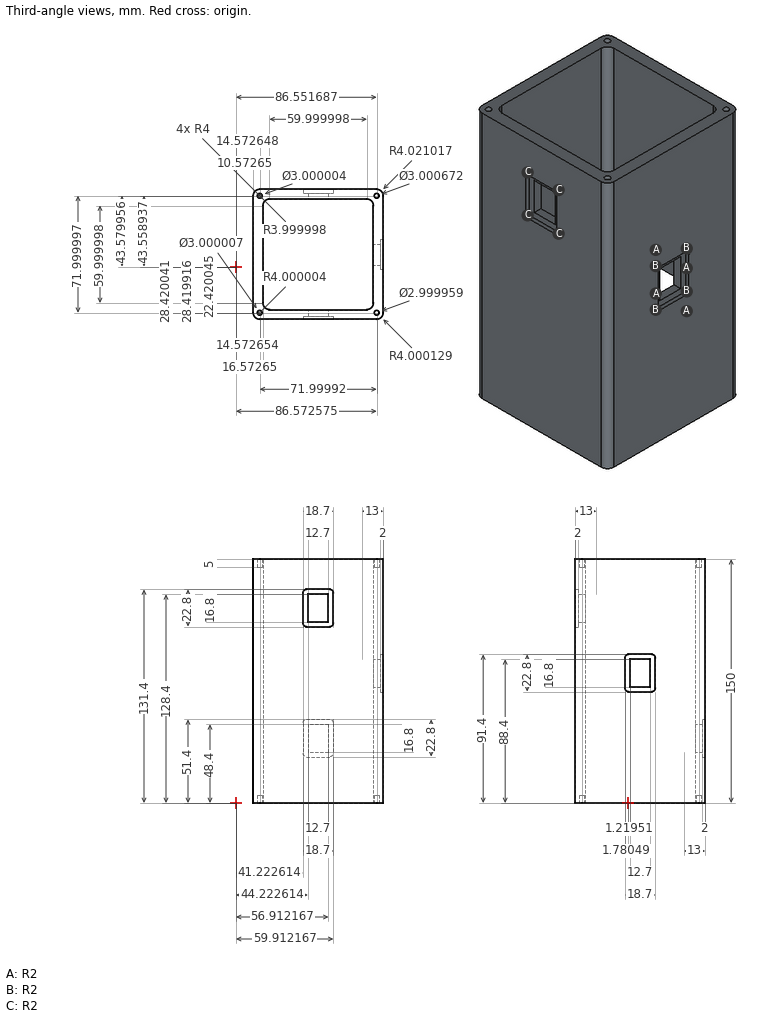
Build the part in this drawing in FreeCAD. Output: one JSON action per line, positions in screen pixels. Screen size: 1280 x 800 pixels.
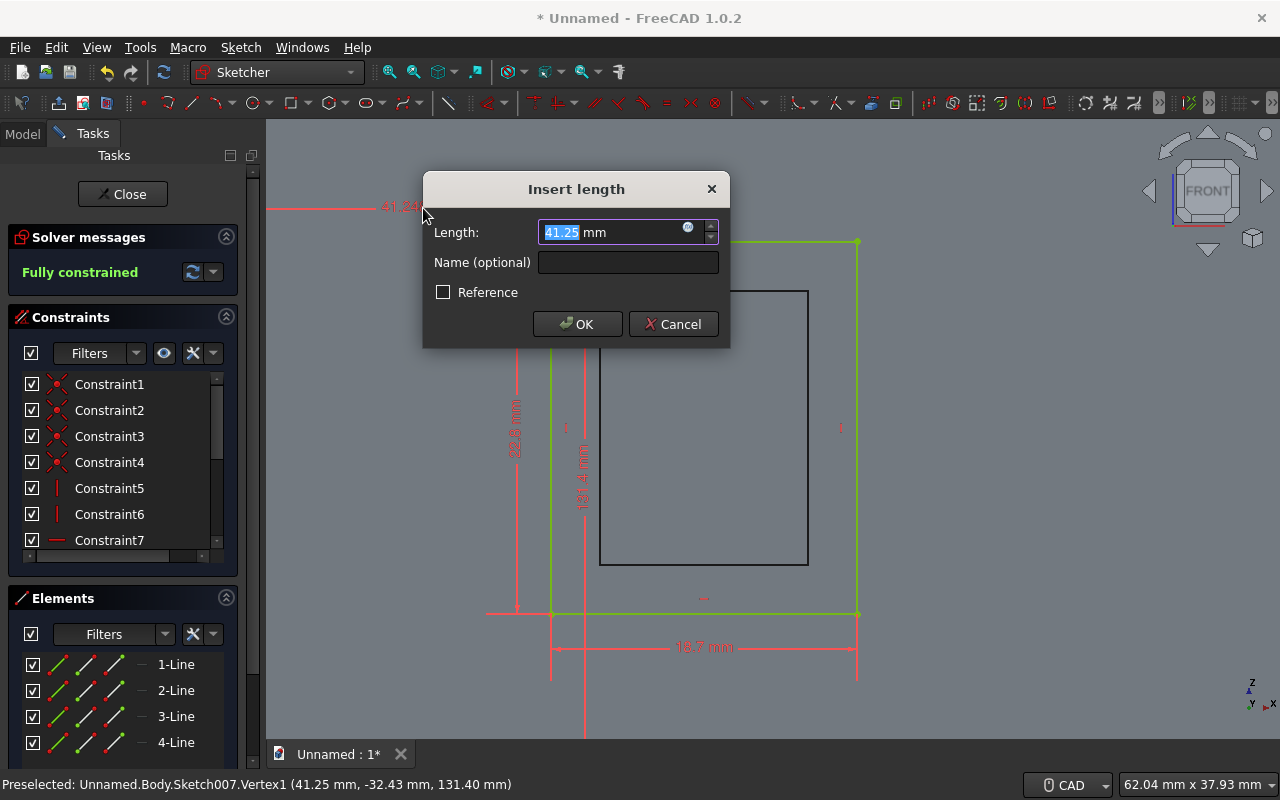
{"action": "type", "text": "41.222614"}
{"action": "key", "text": "Return"}
{"action": "key", "text": "Escape"}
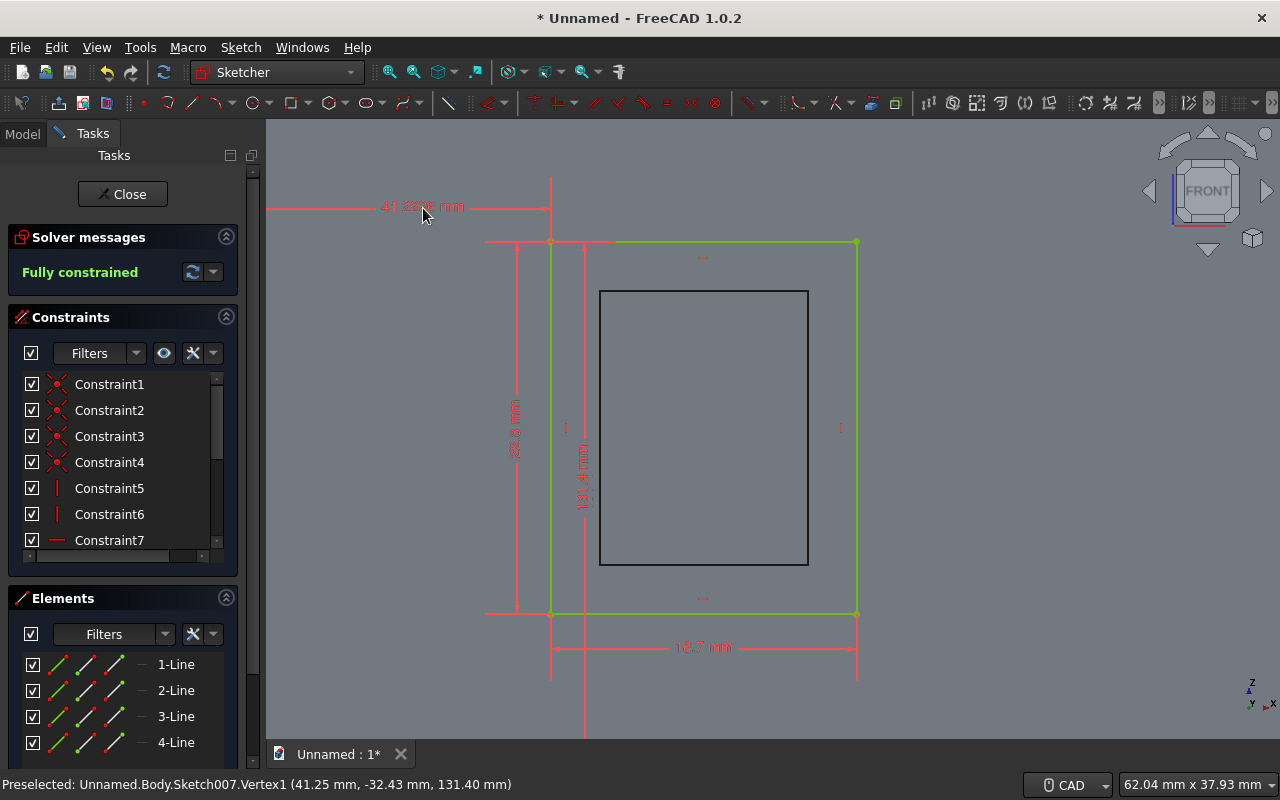
{"action": "left_click", "coordinate": [123, 194]}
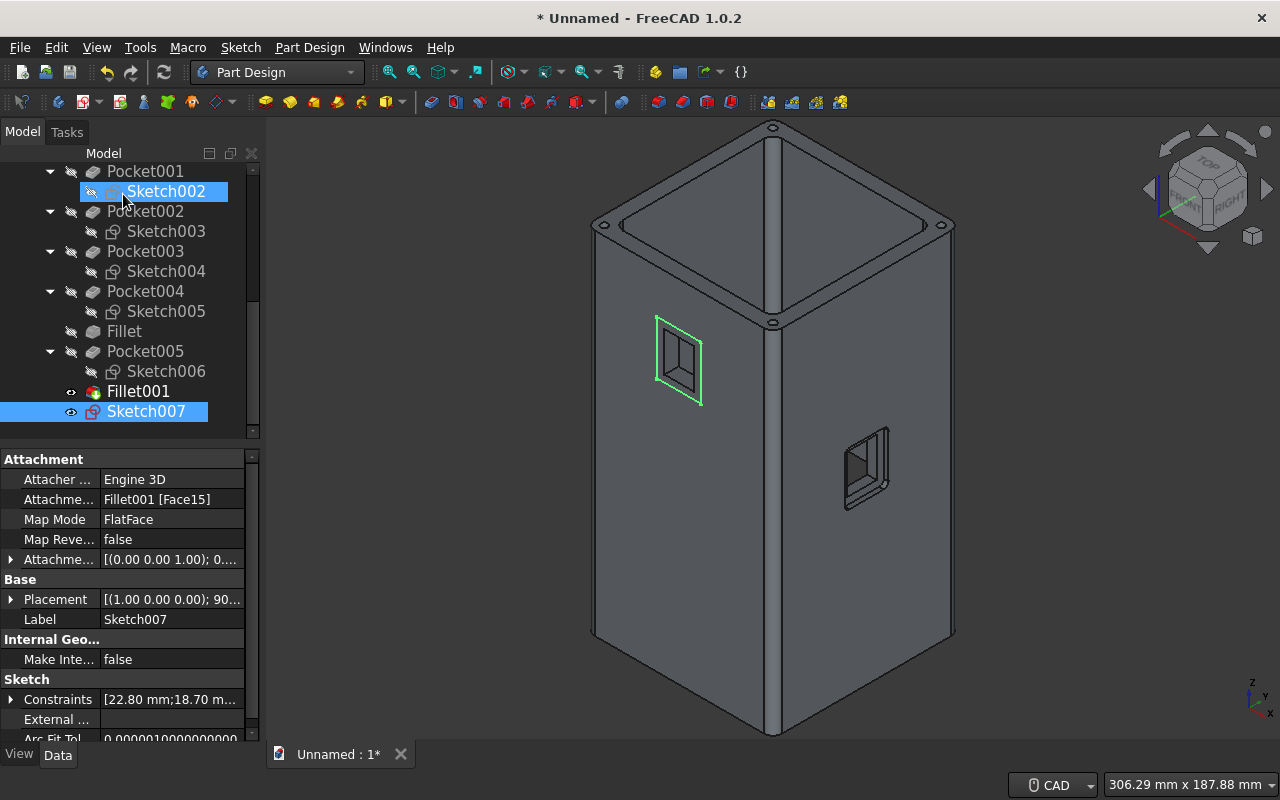
{"action": "left_click", "coordinate": [432, 102]}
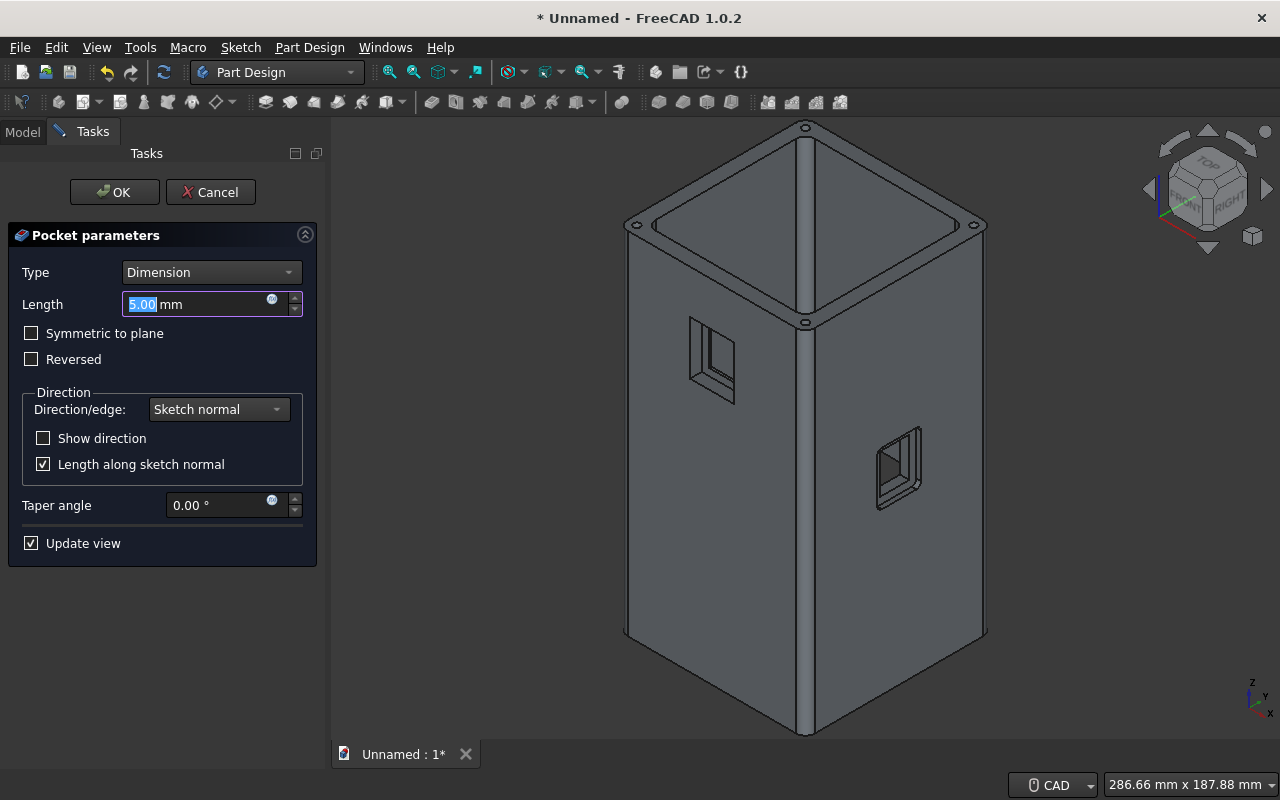
{"action": "type", "text": "2"}
{"action": "key", "text": "Tab"}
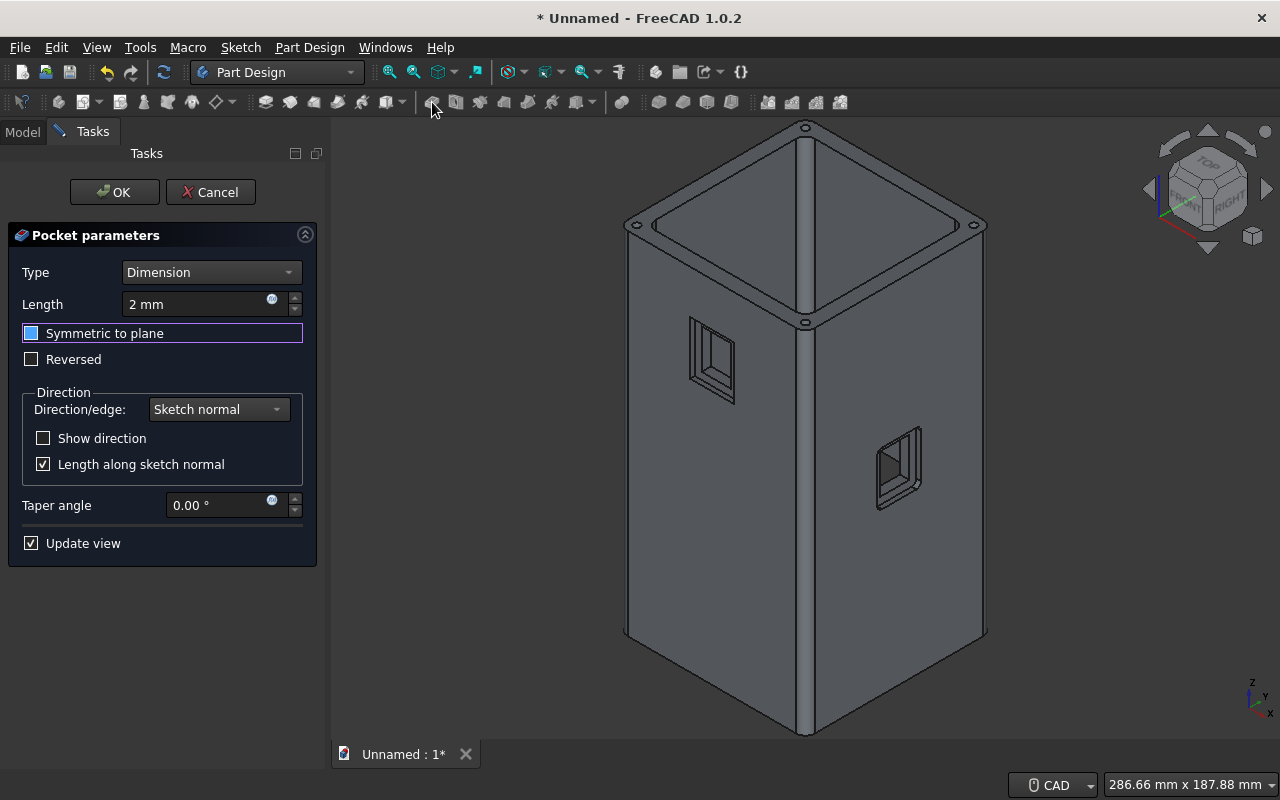
{"action": "left_click", "coordinate": [115, 192]}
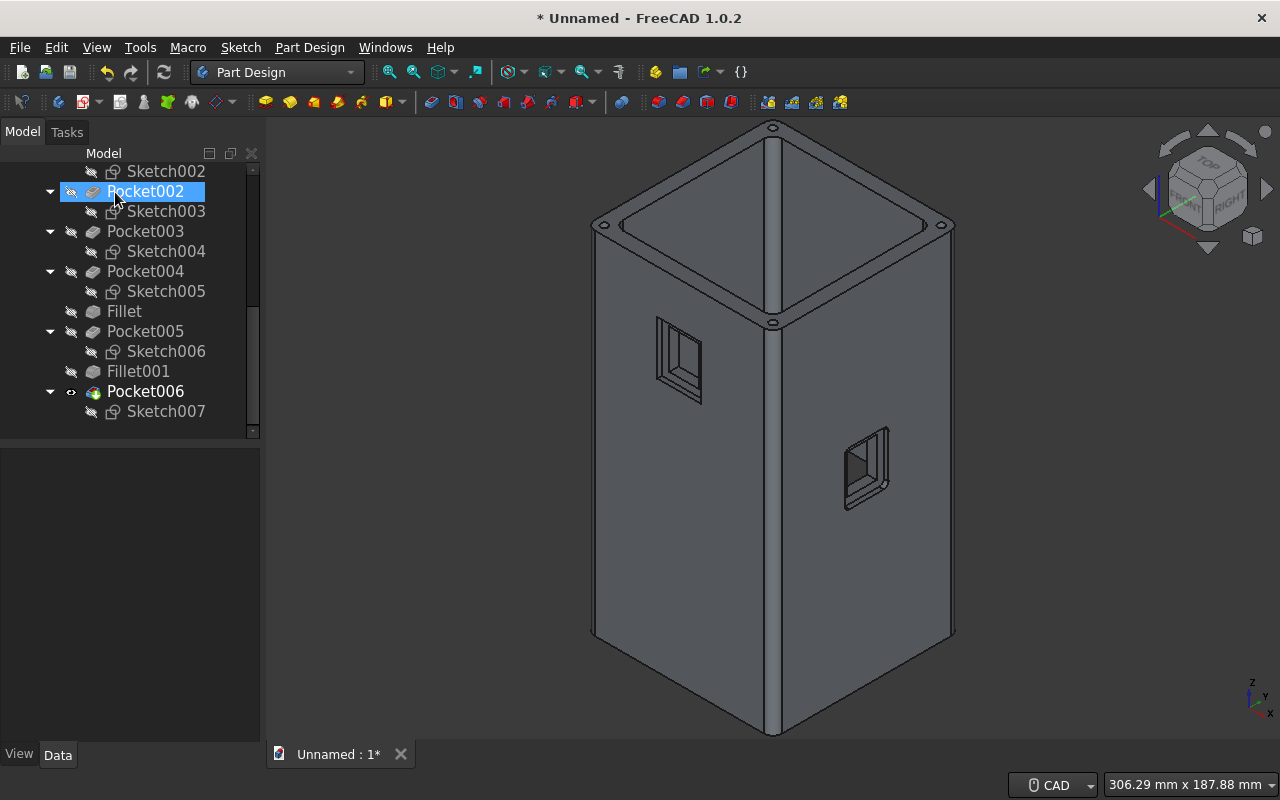
{"action": "left_click", "coordinate": [390, 72]}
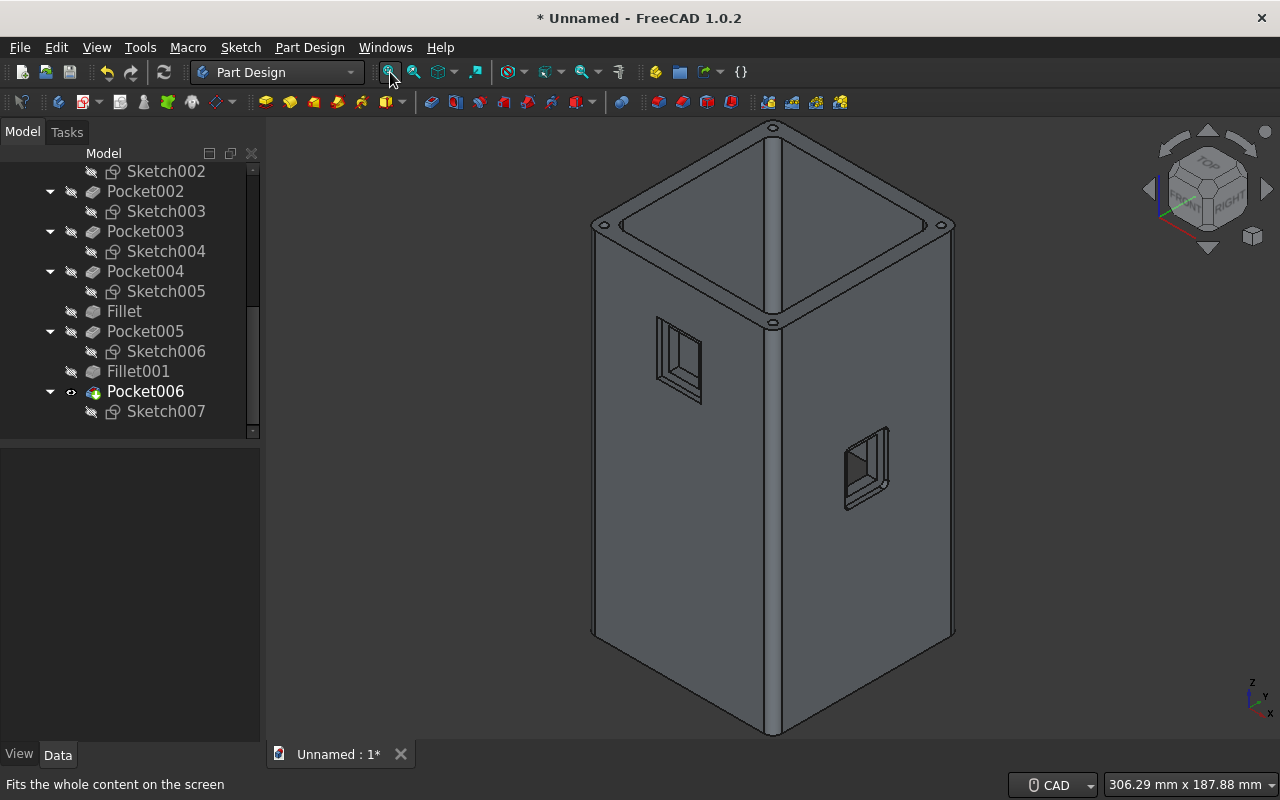
{"action": "scroll", "coordinate": [660, 376], "scroll_direction": "up", "scroll_amount": 9}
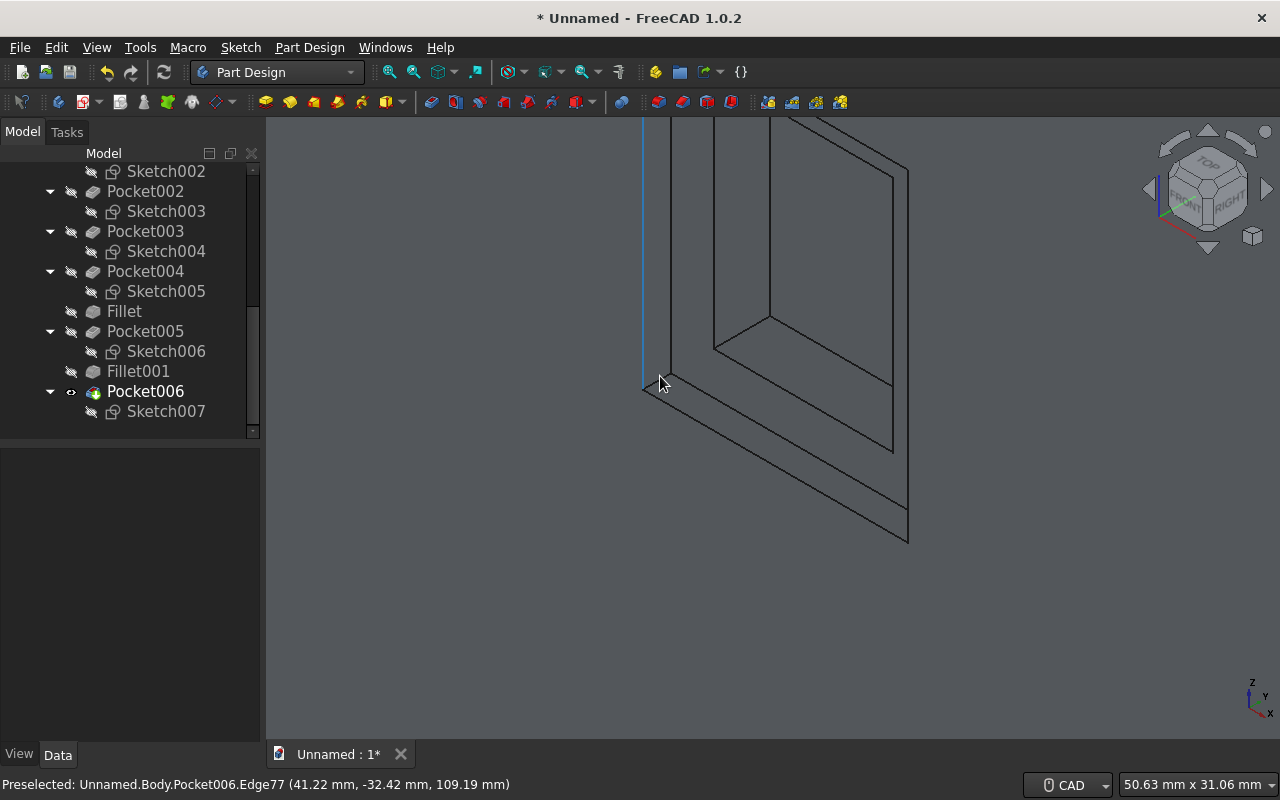
{"action": "left_click", "coordinate": [390, 72]}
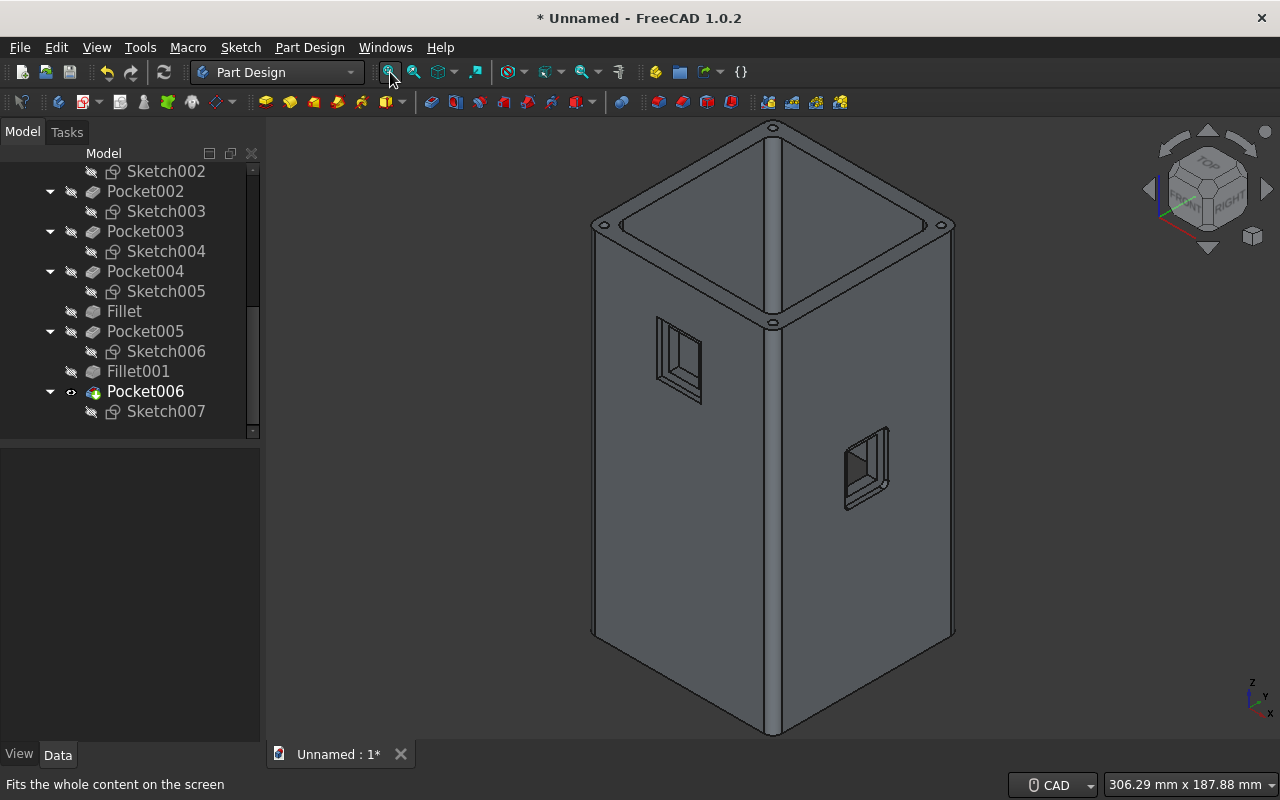
{"action": "key", "text": "2"}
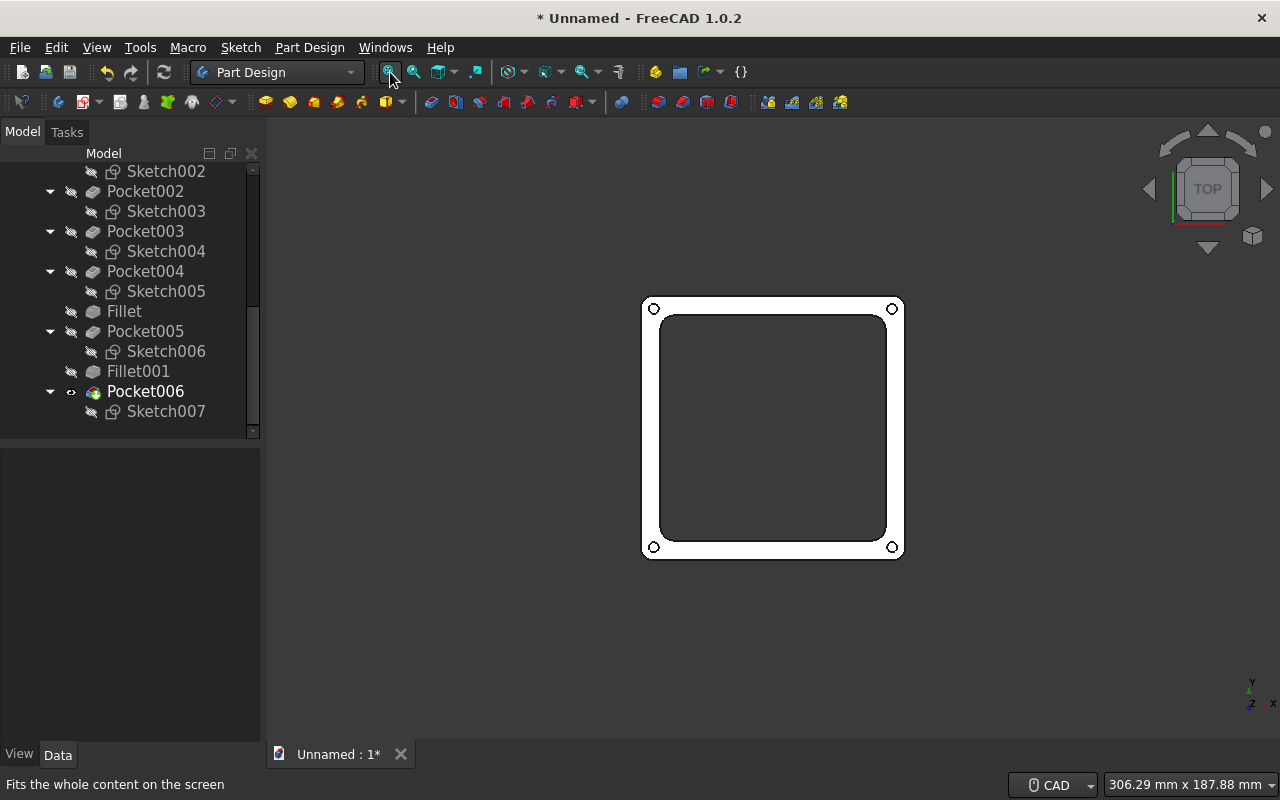
{"action": "left_click", "coordinate": [390, 72]}